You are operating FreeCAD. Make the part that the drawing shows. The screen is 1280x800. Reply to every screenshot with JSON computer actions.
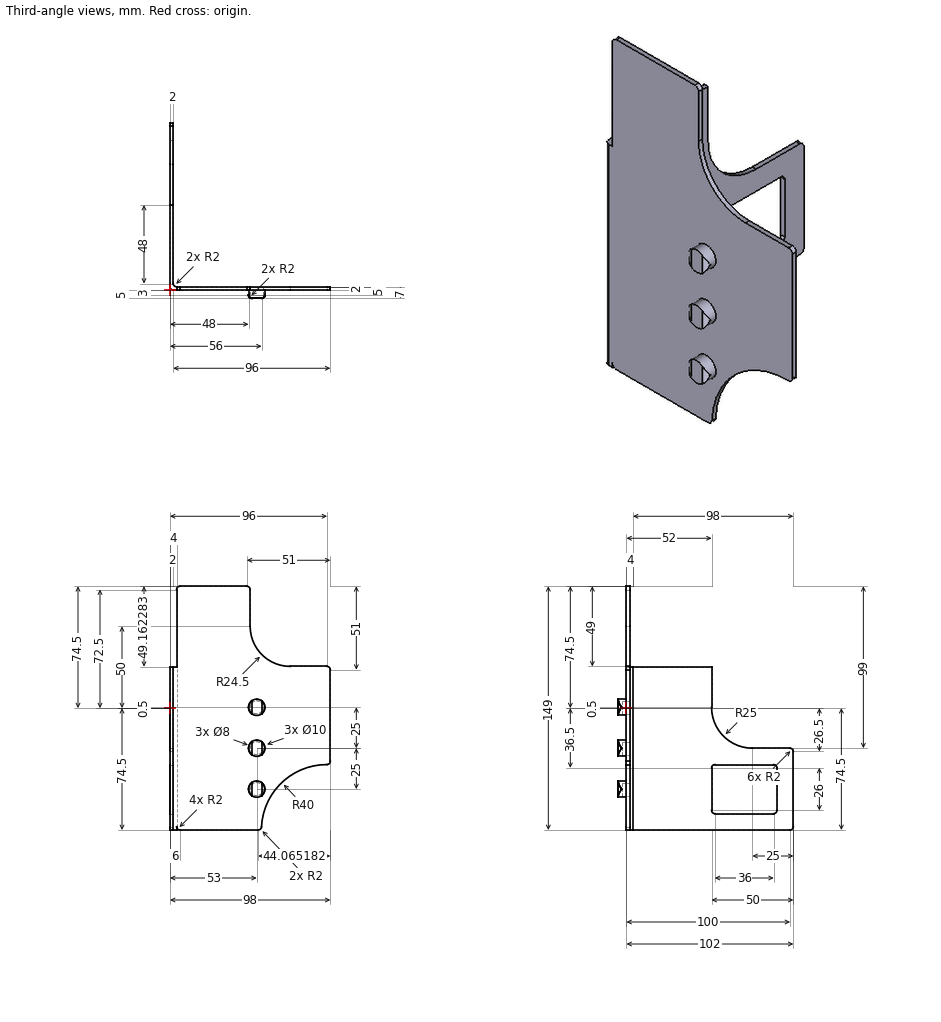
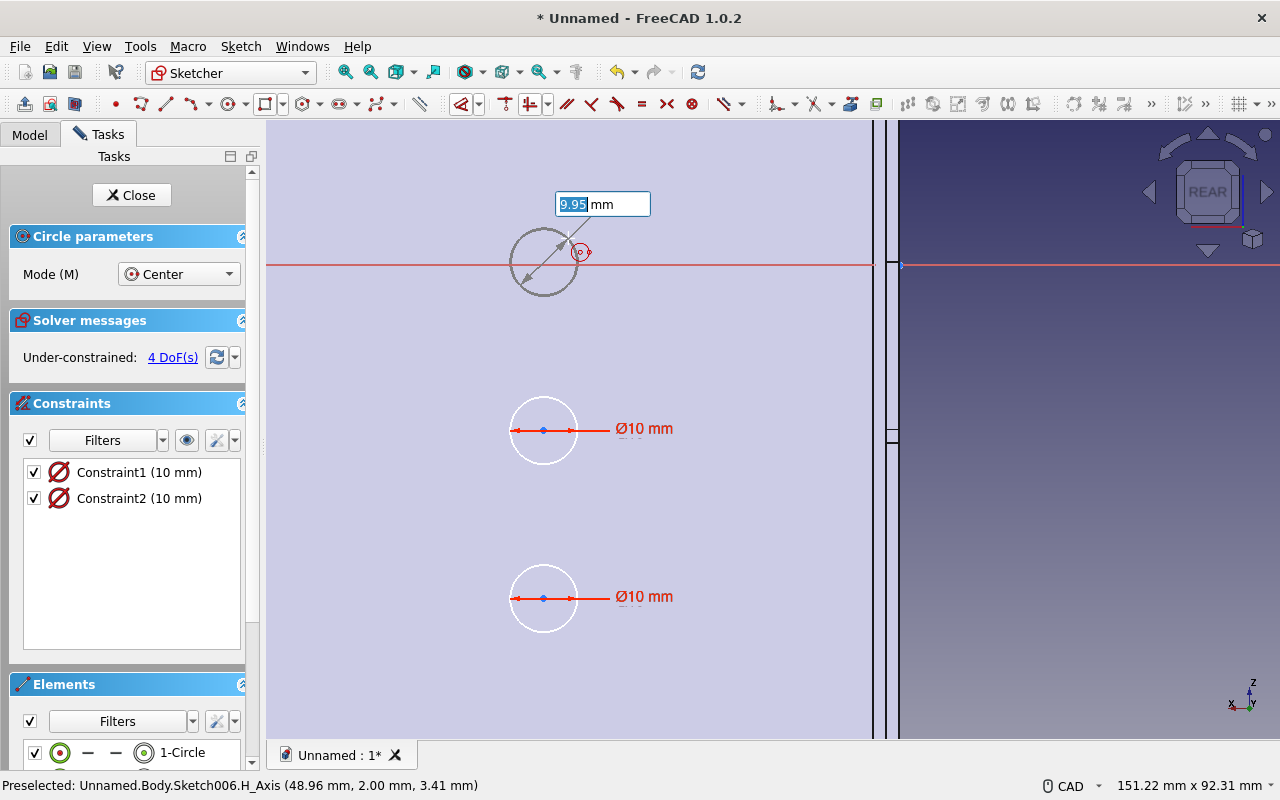
{"action": "type", "text": "10"}
{"action": "key", "text": "Return"}
{"action": "key", "text": "Escape"}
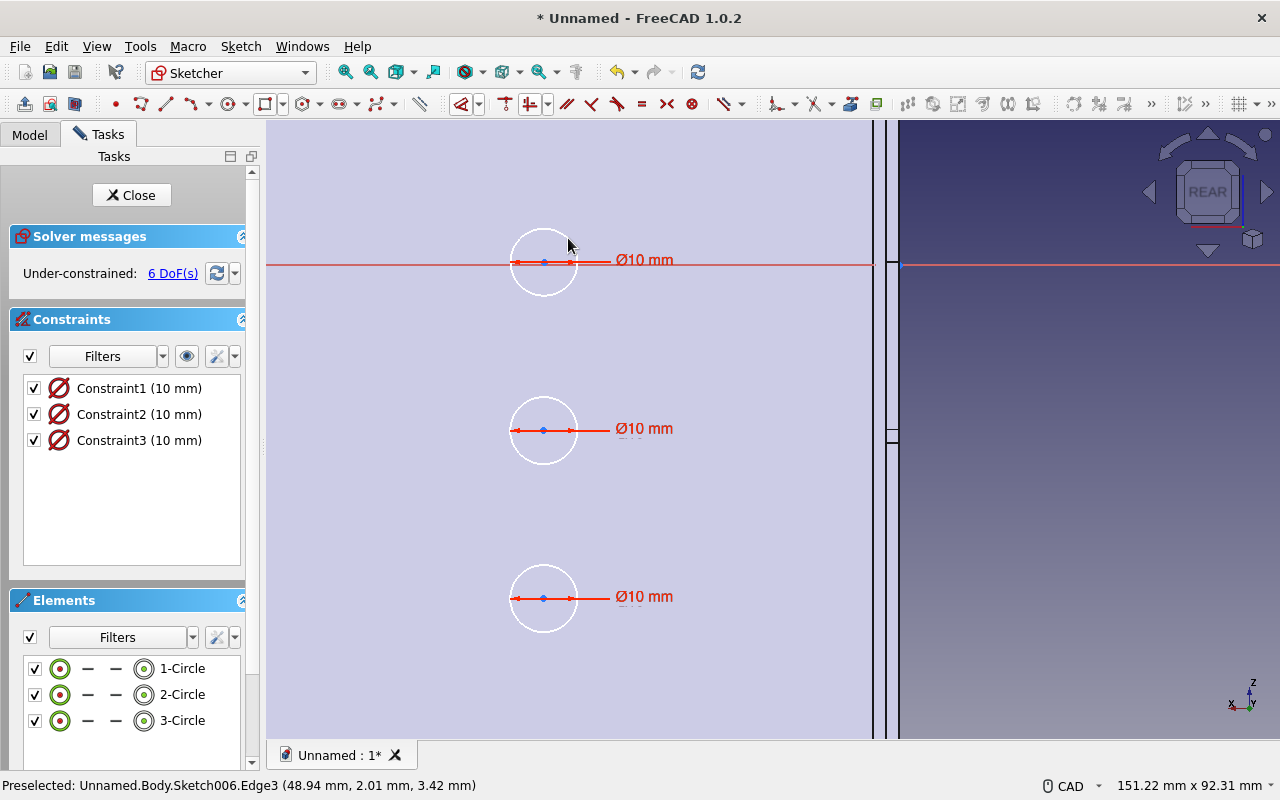
{"action": "left_click", "coordinate": [544, 431]}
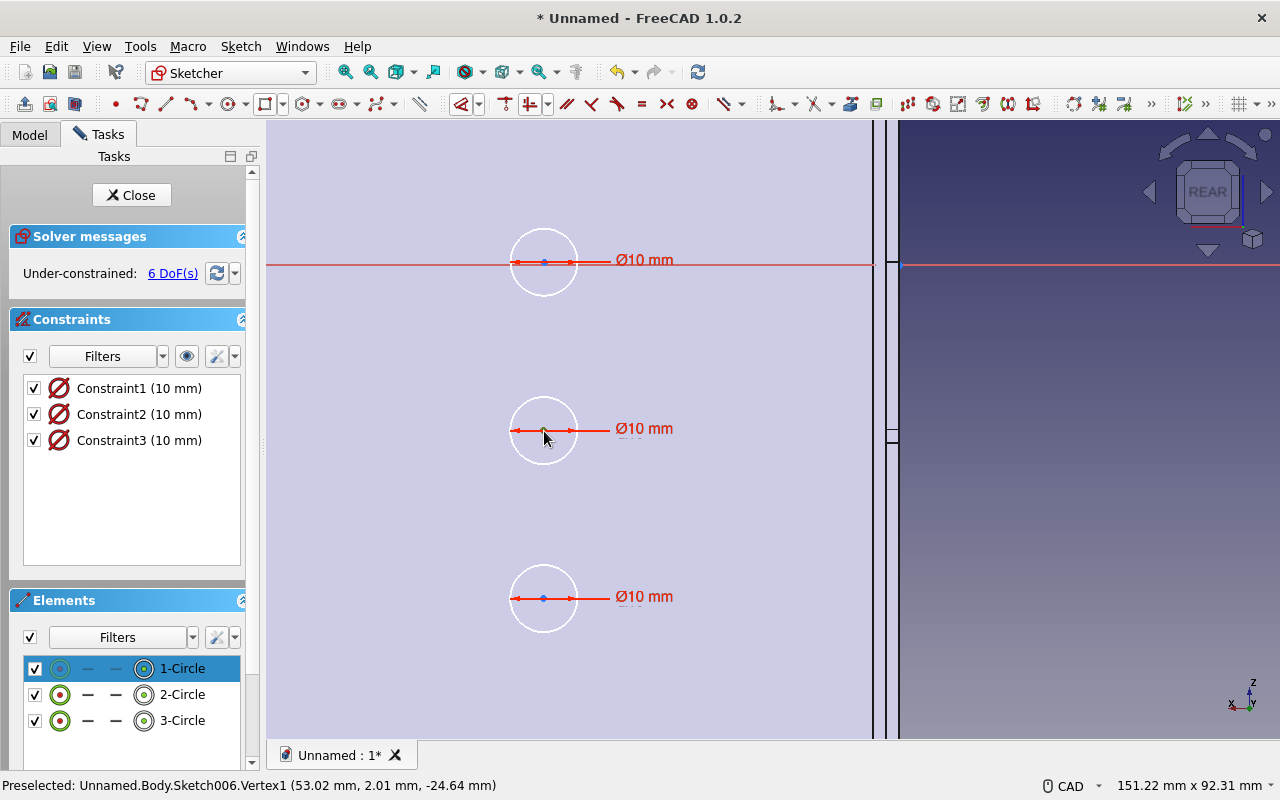
{"action": "left_click", "coordinate": [544, 599]}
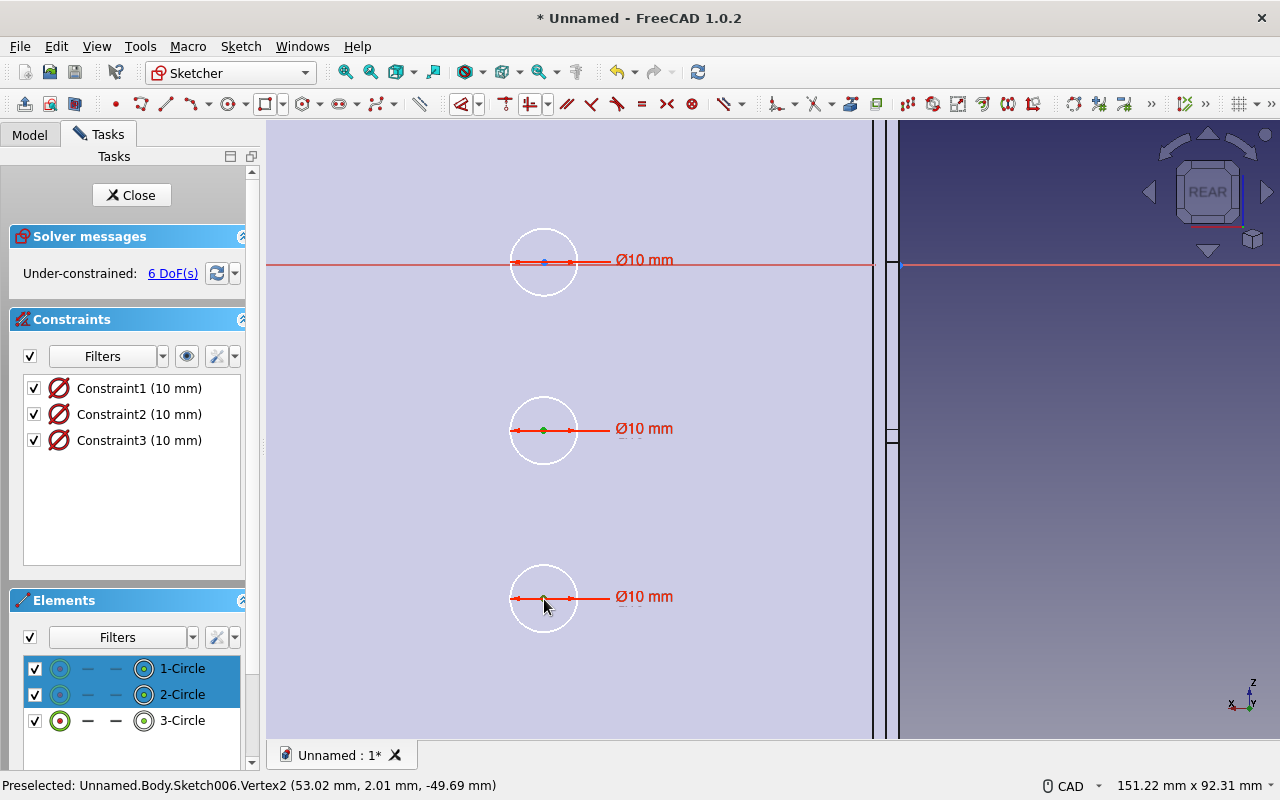
{"action": "left_click", "coordinate": [548, 104]}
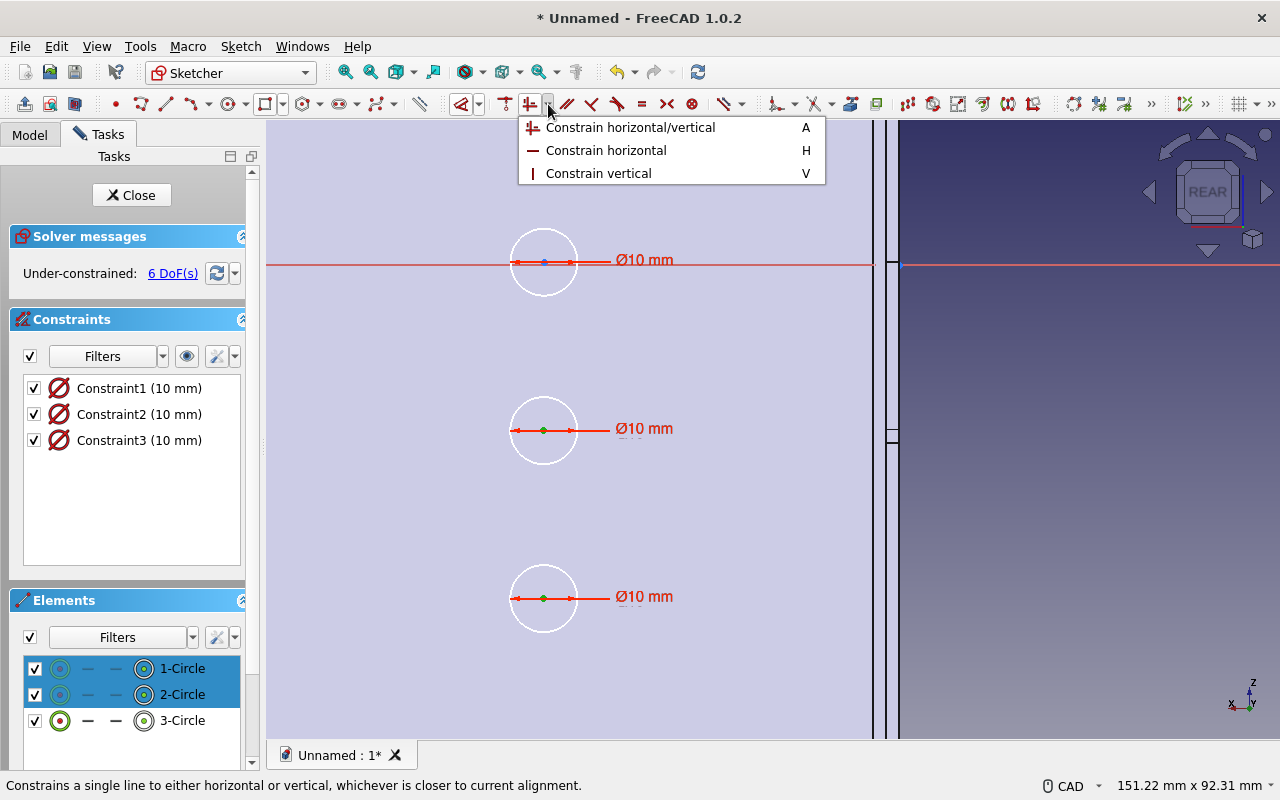
{"action": "left_click", "coordinate": [672, 174]}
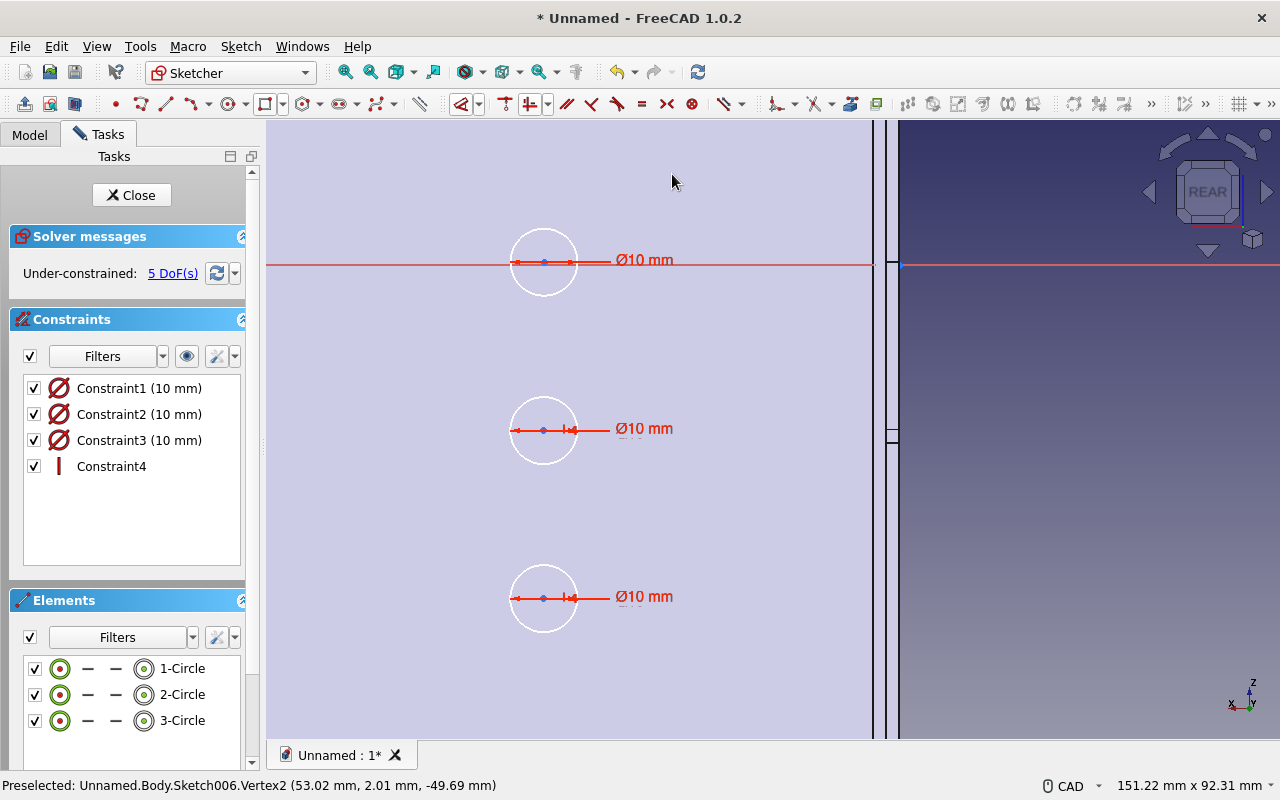
{"action": "left_click", "coordinate": [544, 431]}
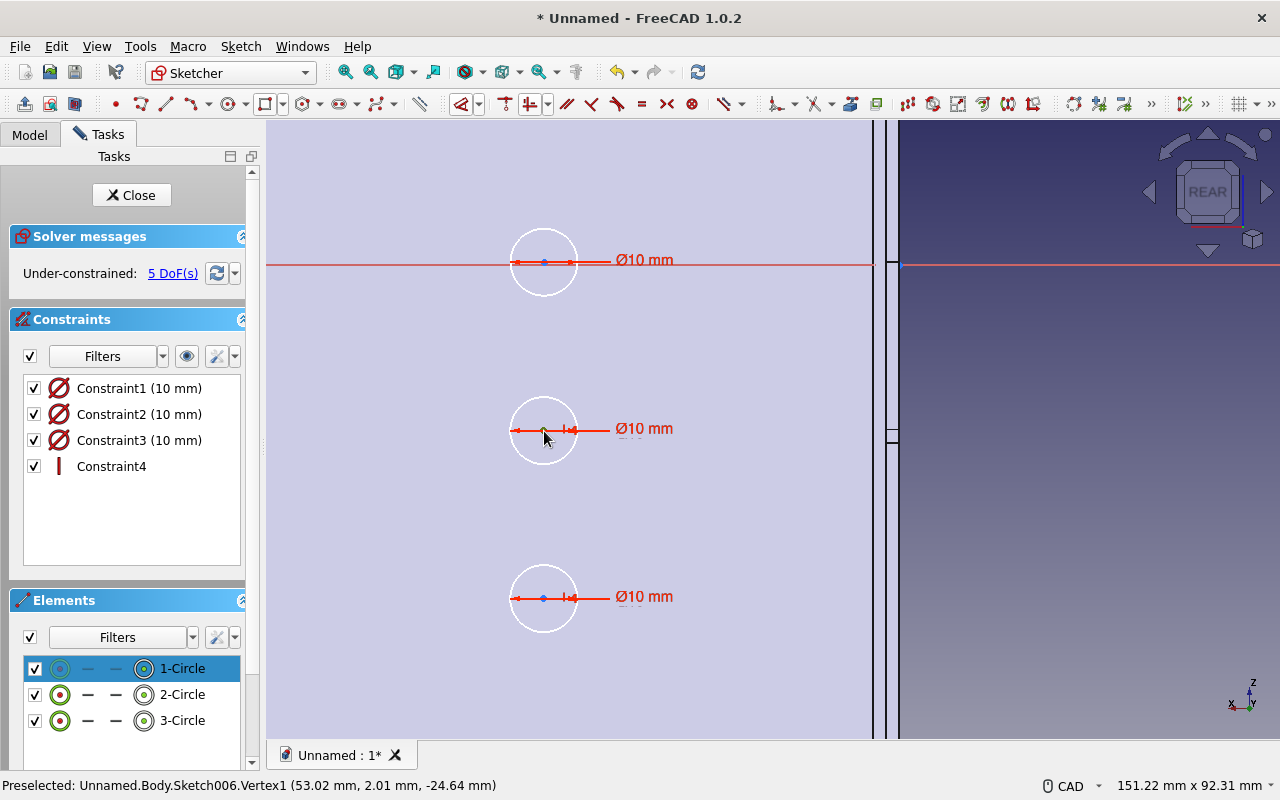
{"action": "left_click", "coordinate": [544, 262]}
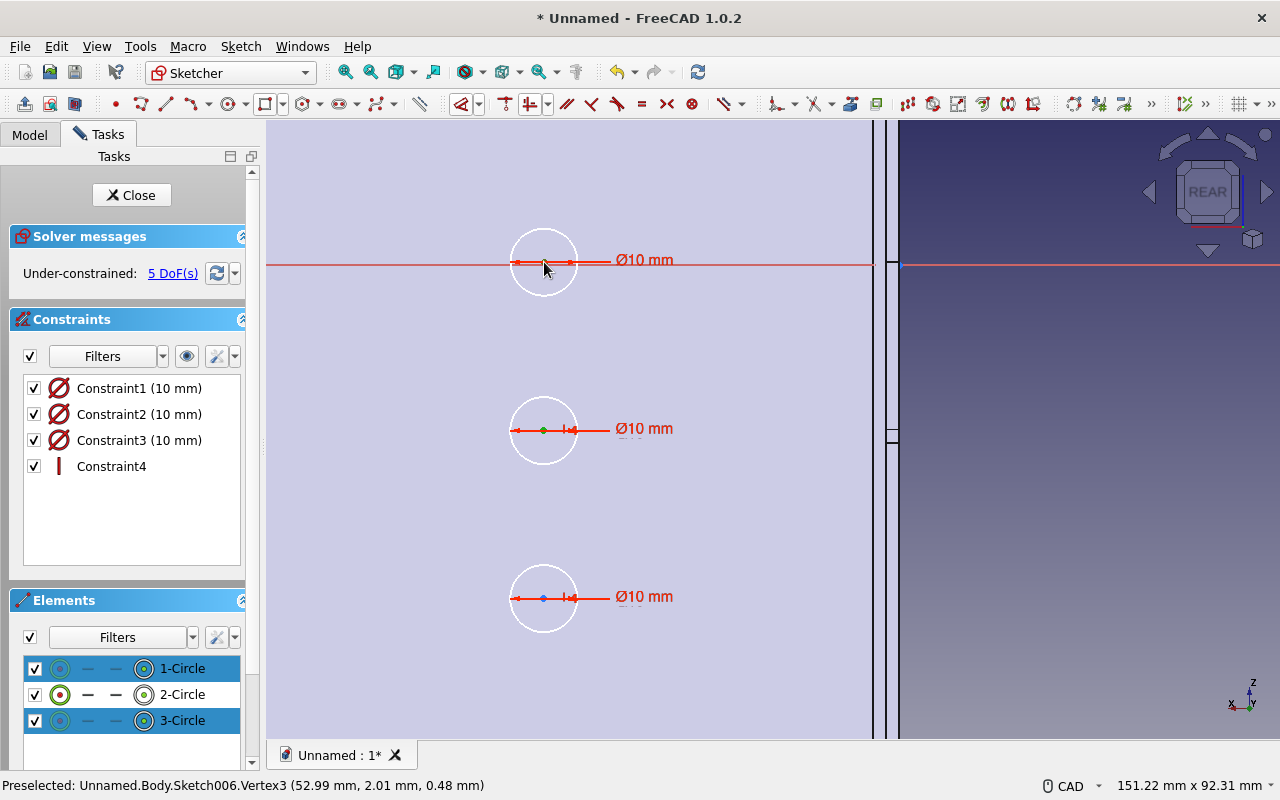
{"action": "key", "text": "v"}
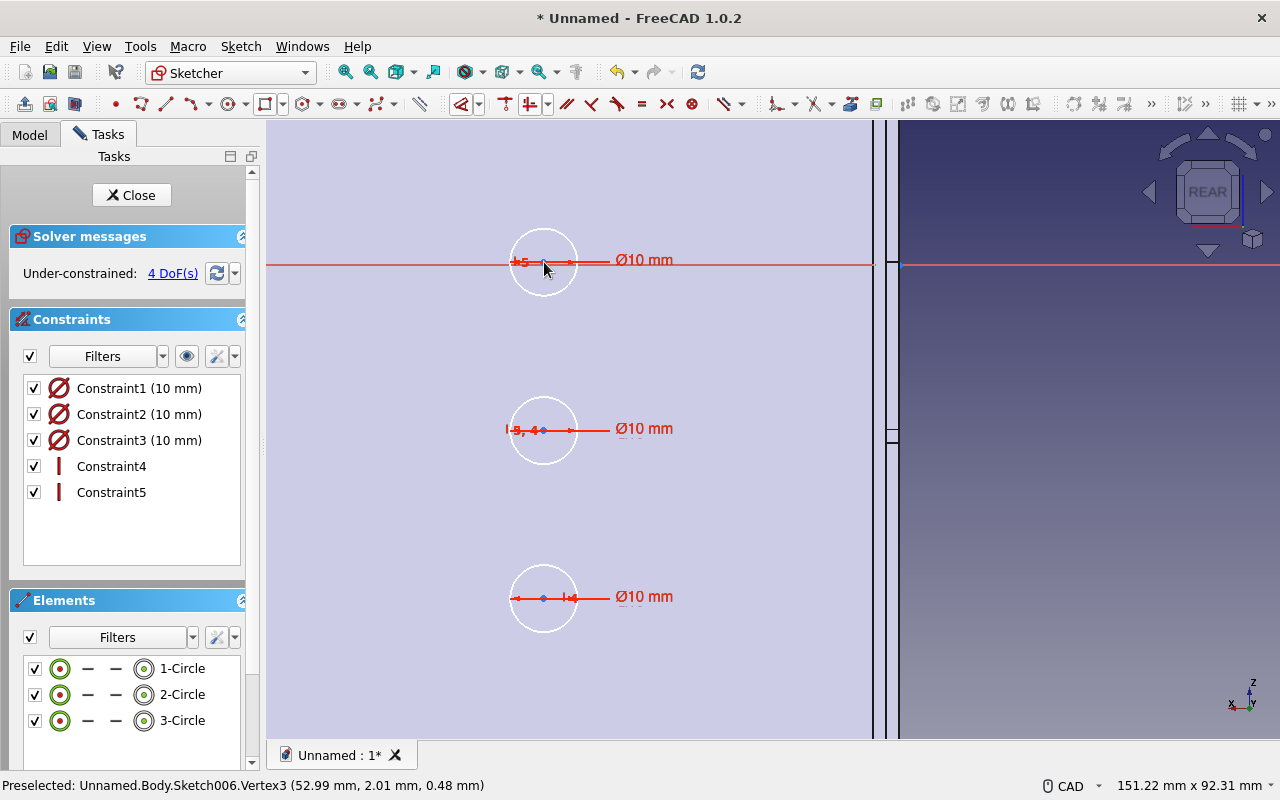
{"action": "left_click", "coordinate": [544, 431]}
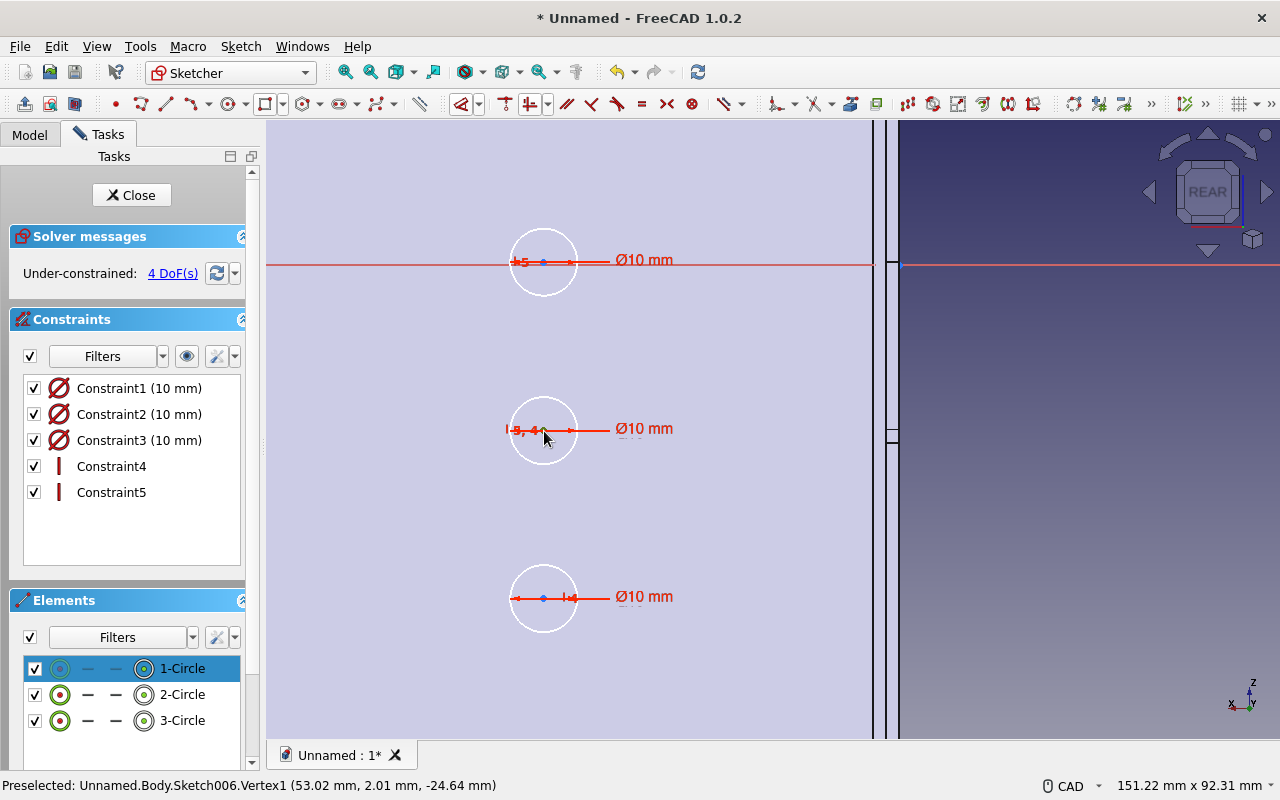
{"action": "key", "text": "l"}